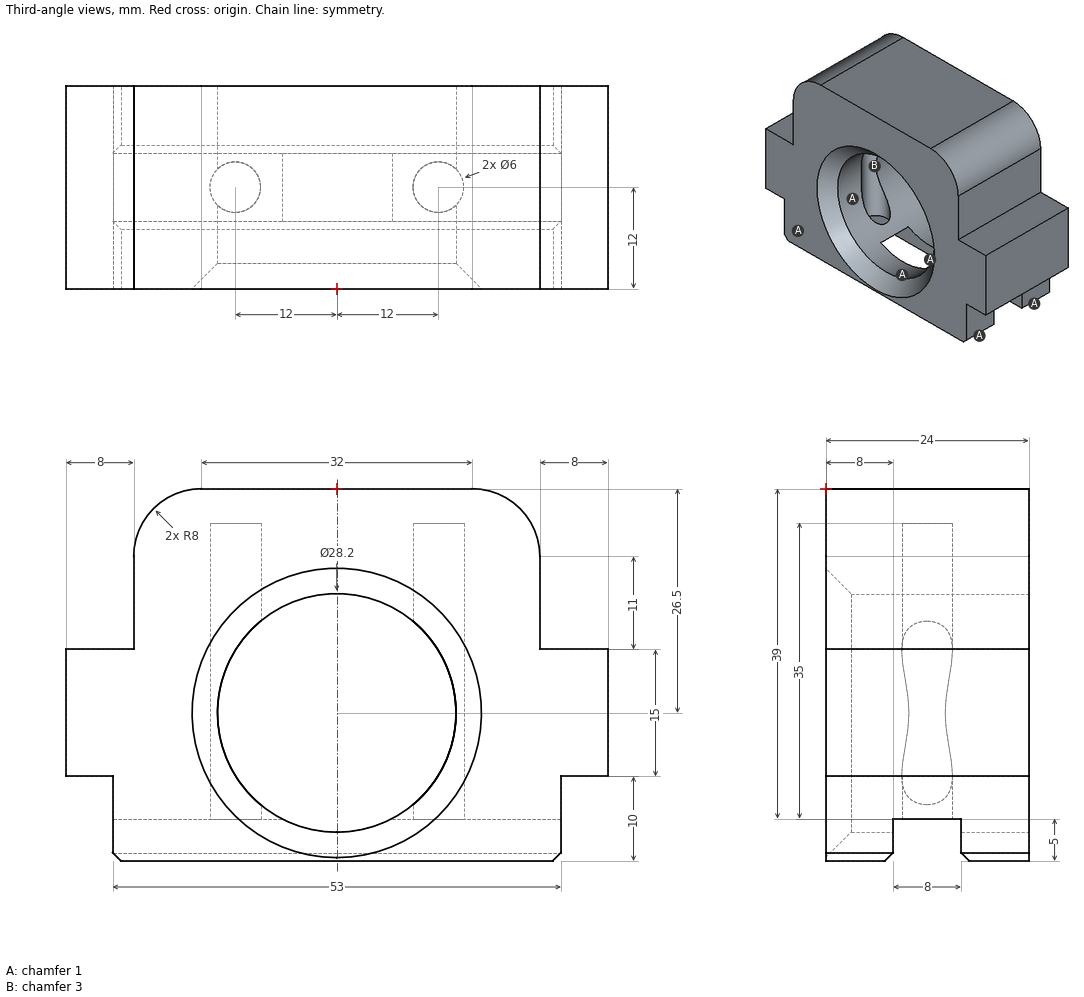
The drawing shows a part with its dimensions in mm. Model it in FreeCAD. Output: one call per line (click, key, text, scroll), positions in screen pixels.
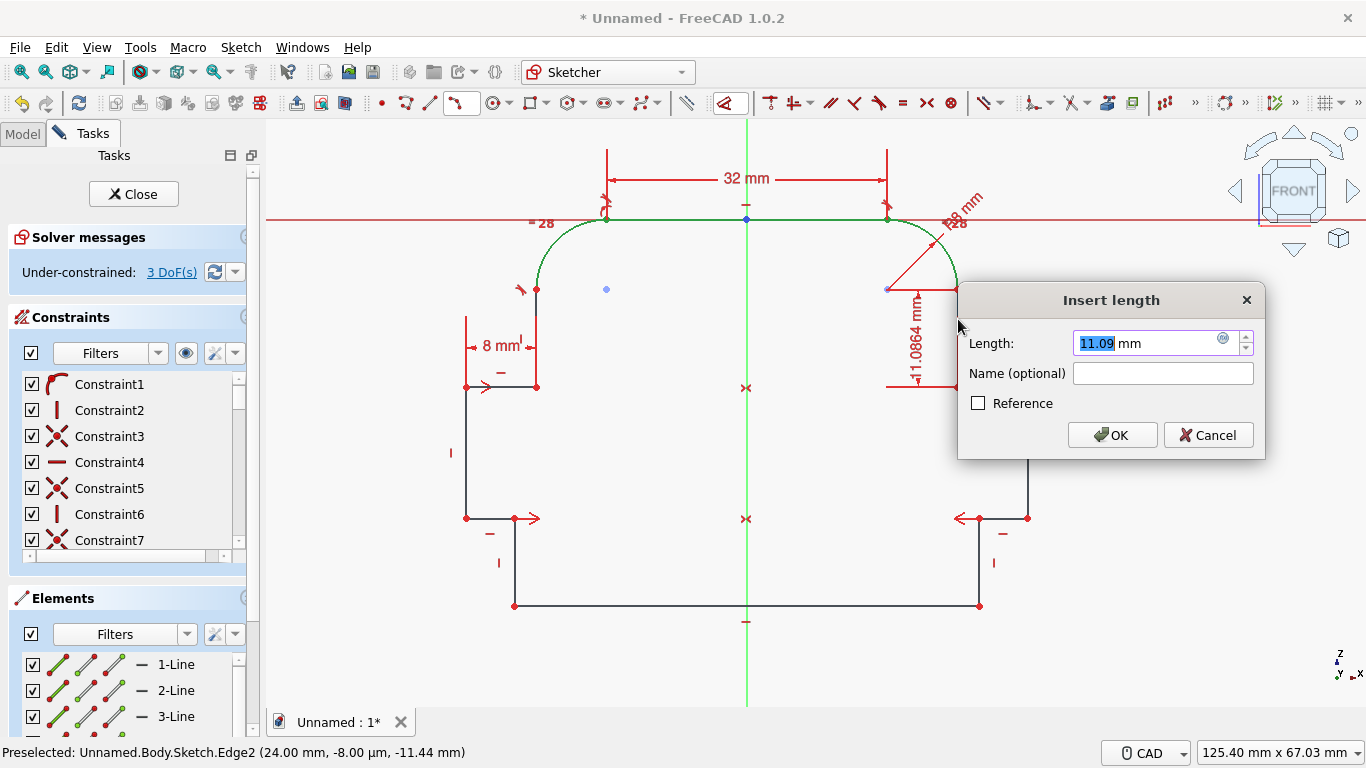
text(11)
key(Return)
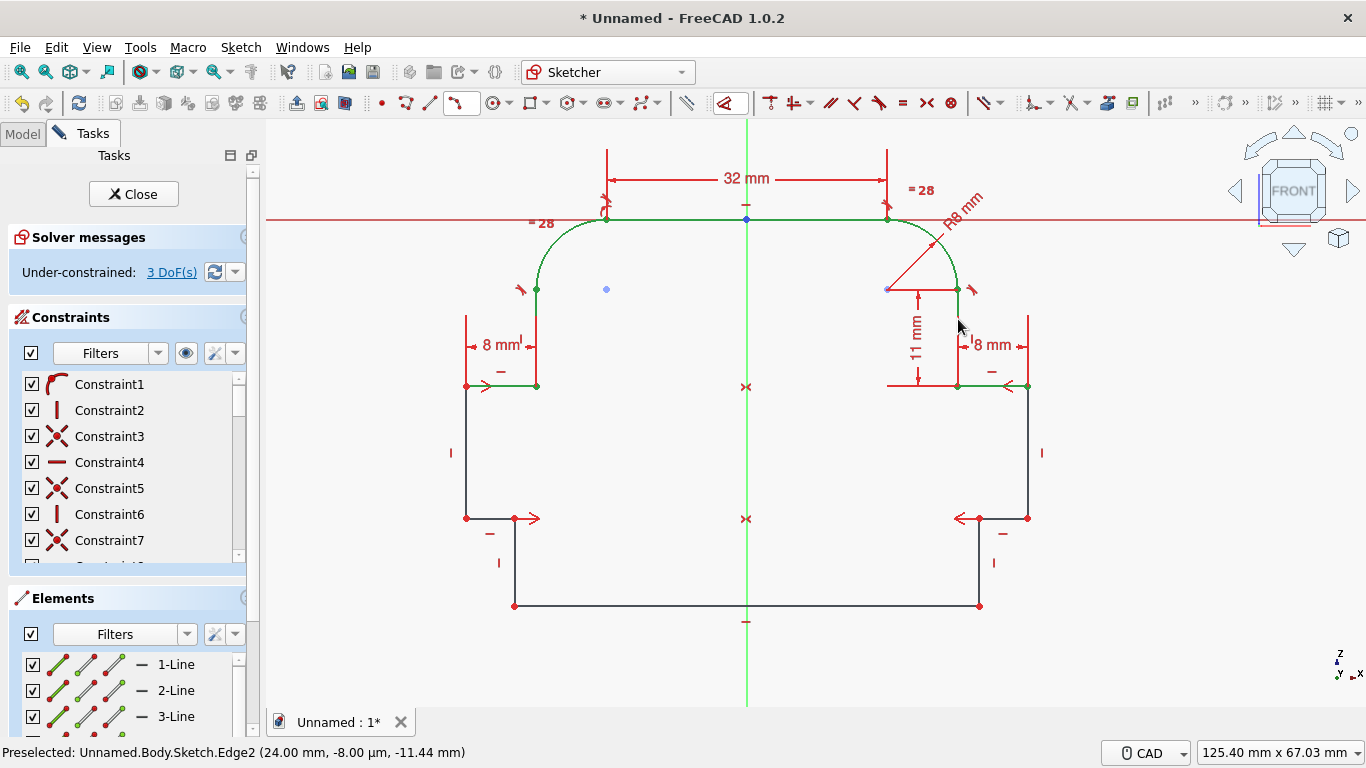
click(1028, 426)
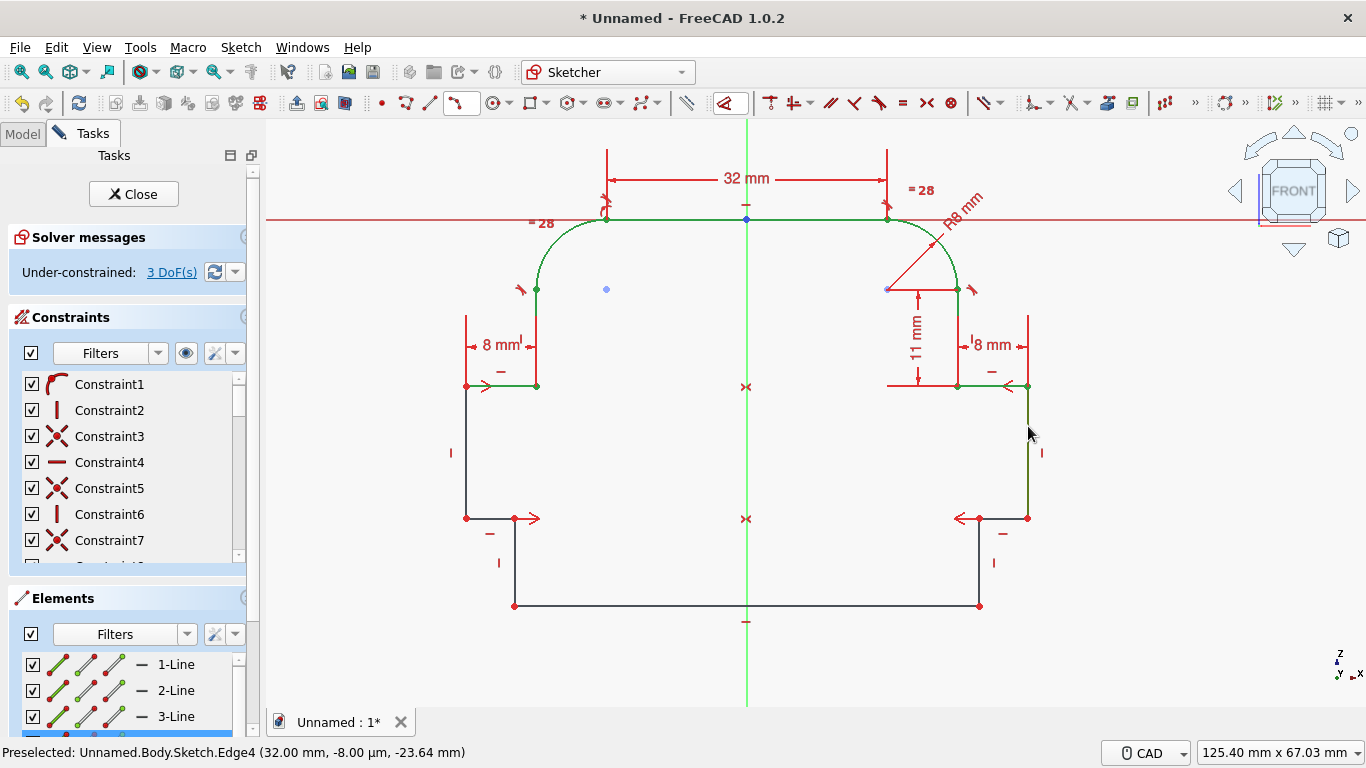
click(742, 104)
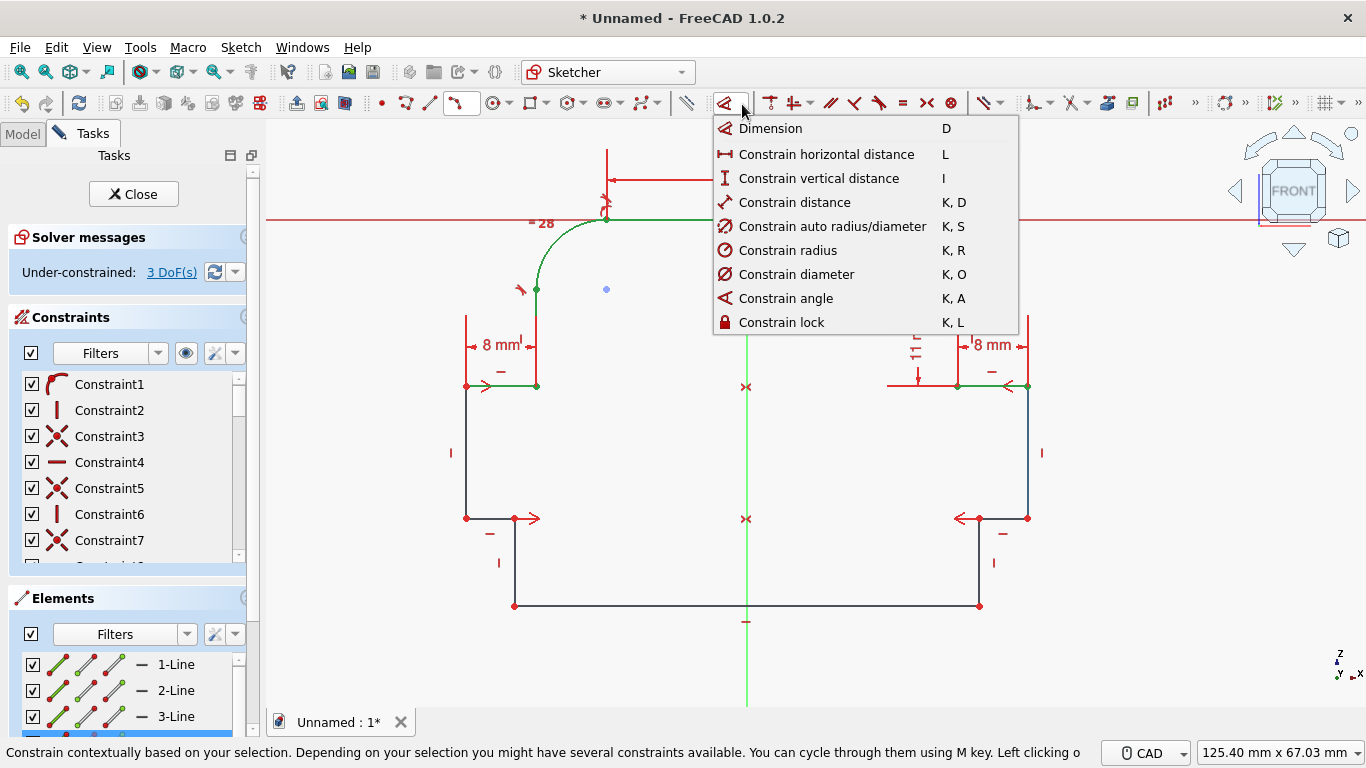
click(866, 178)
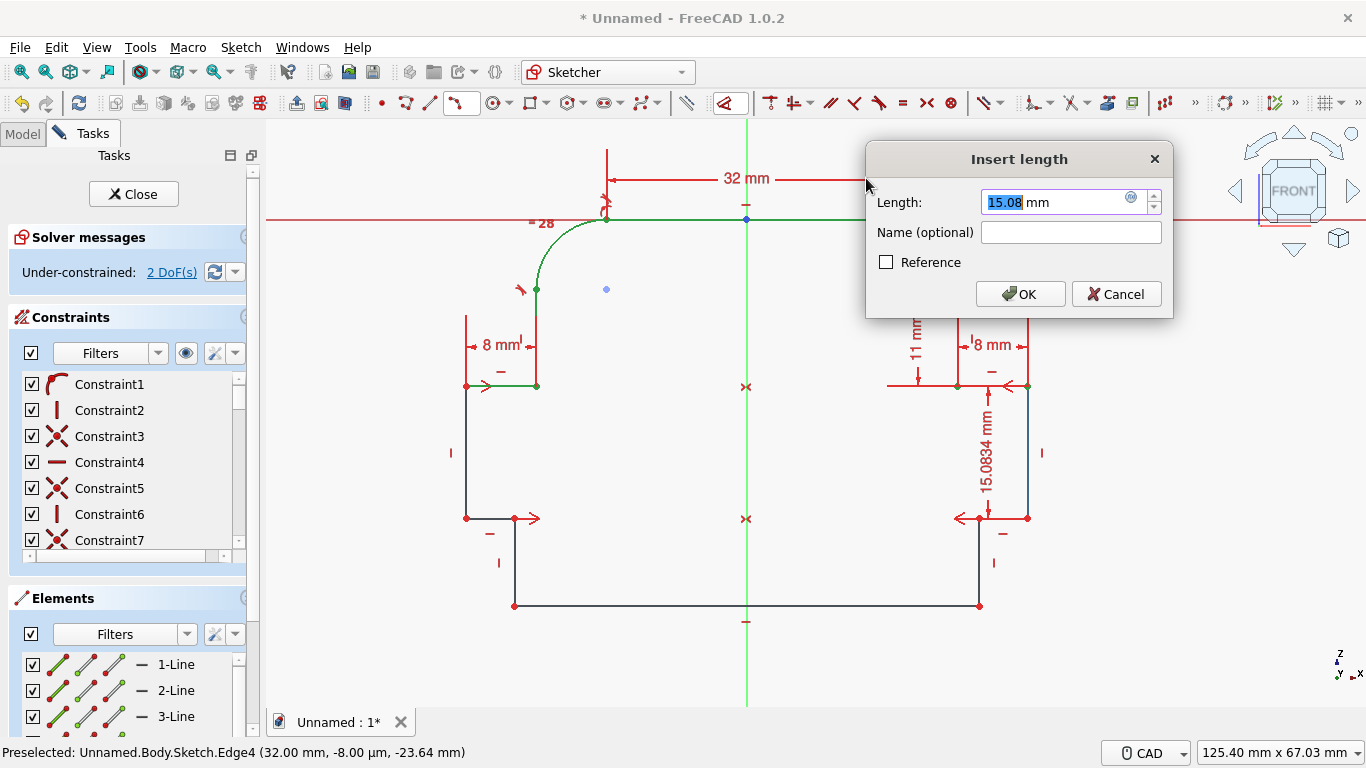
text(15)
key(Return)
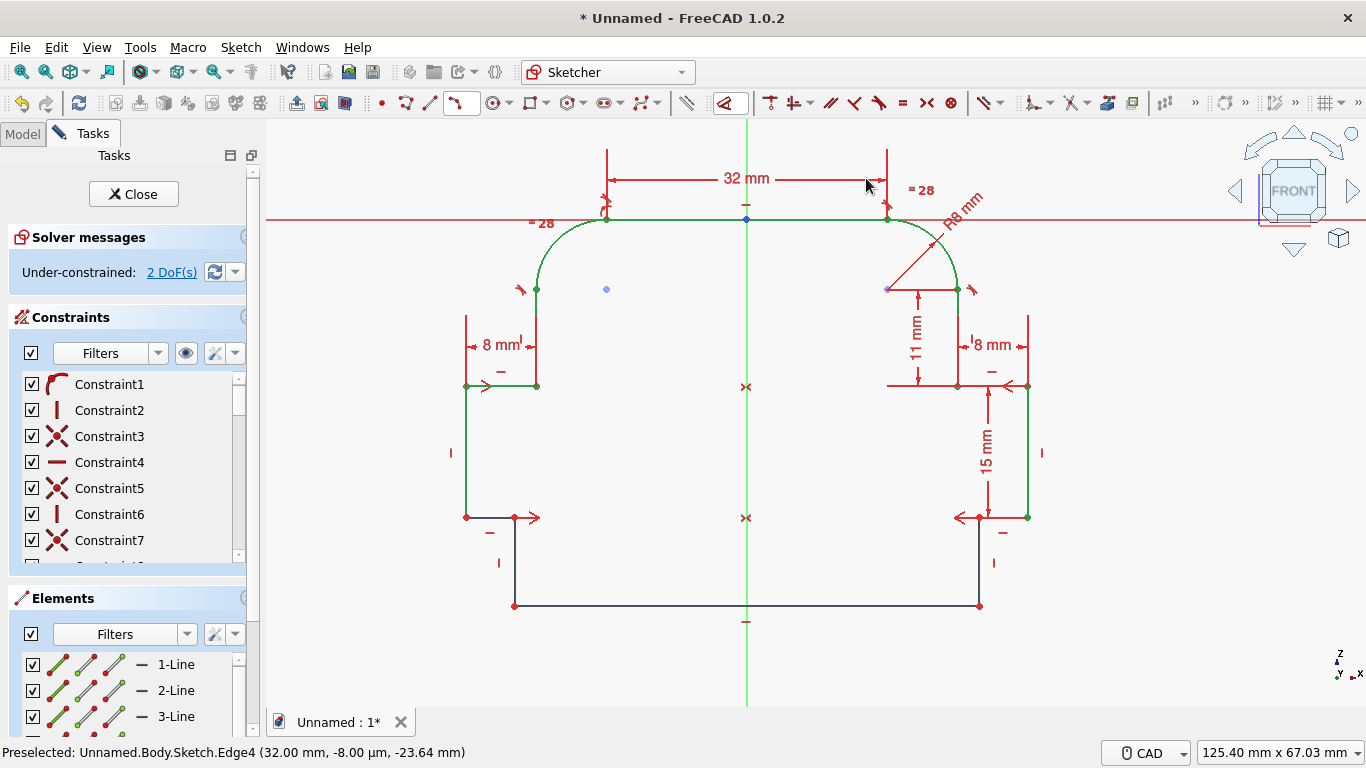
click(979, 544)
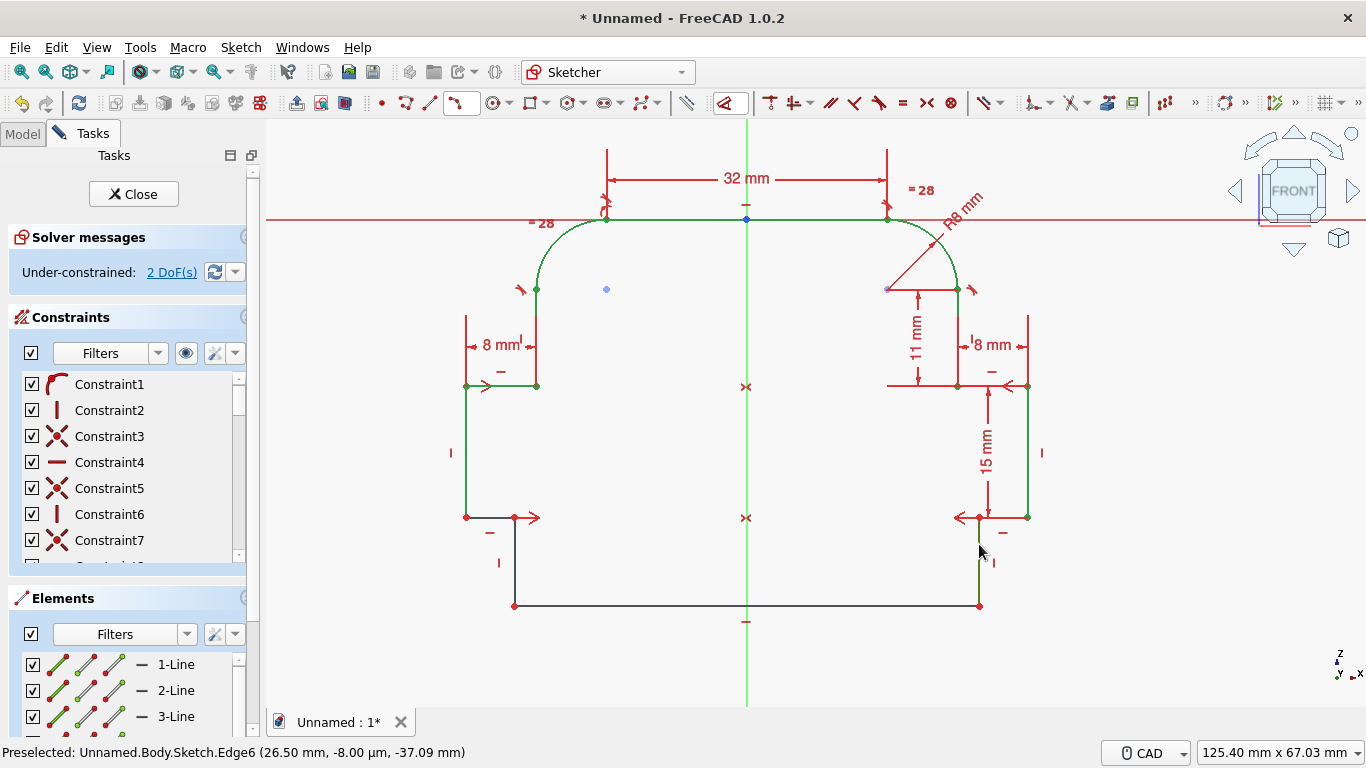
click(742, 104)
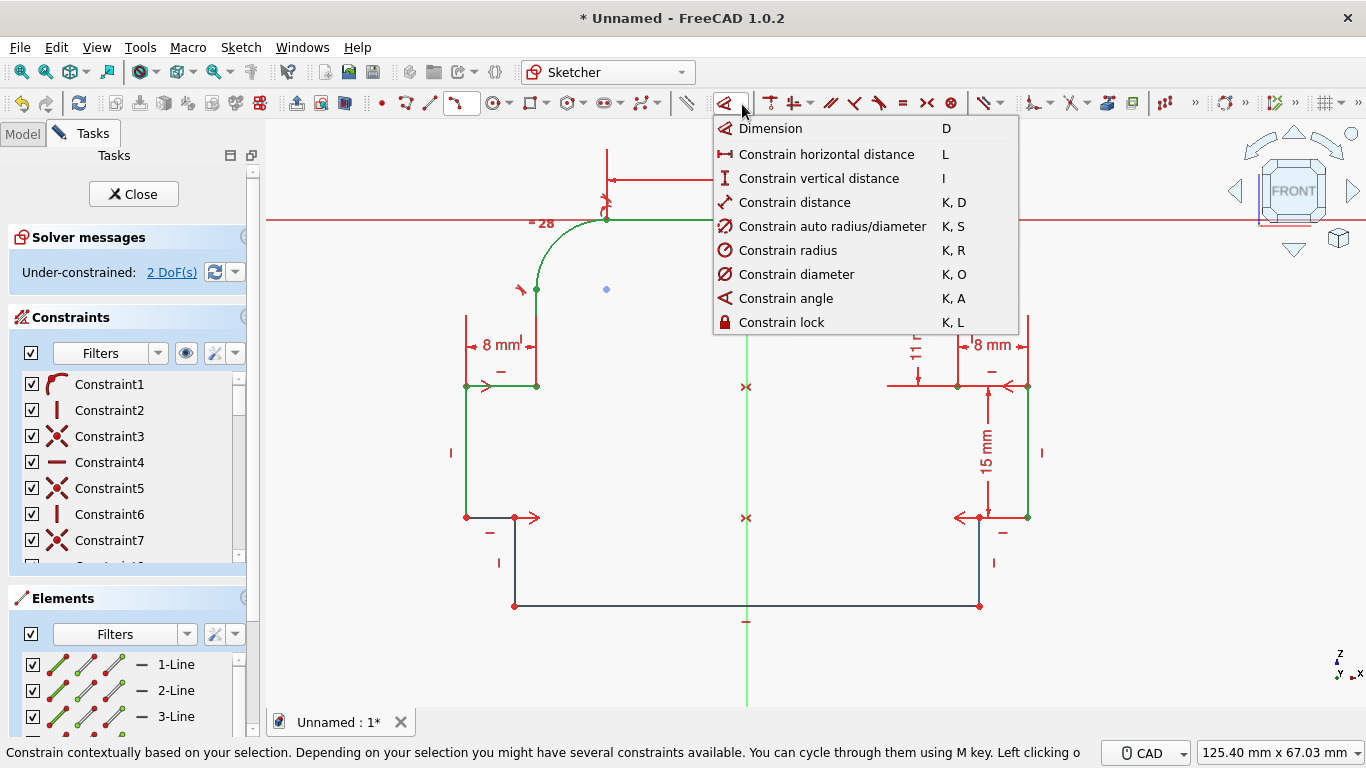
click(866, 178)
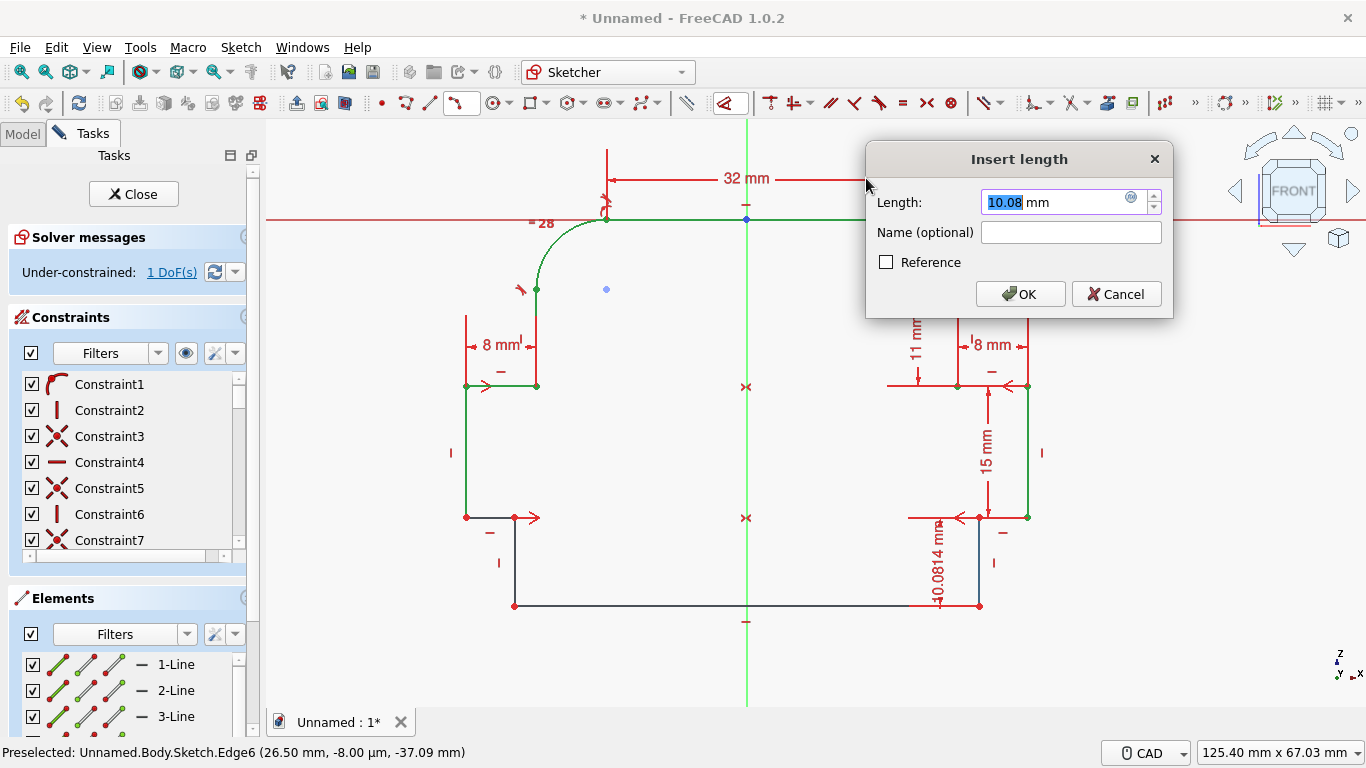
text(10)
key(Return)